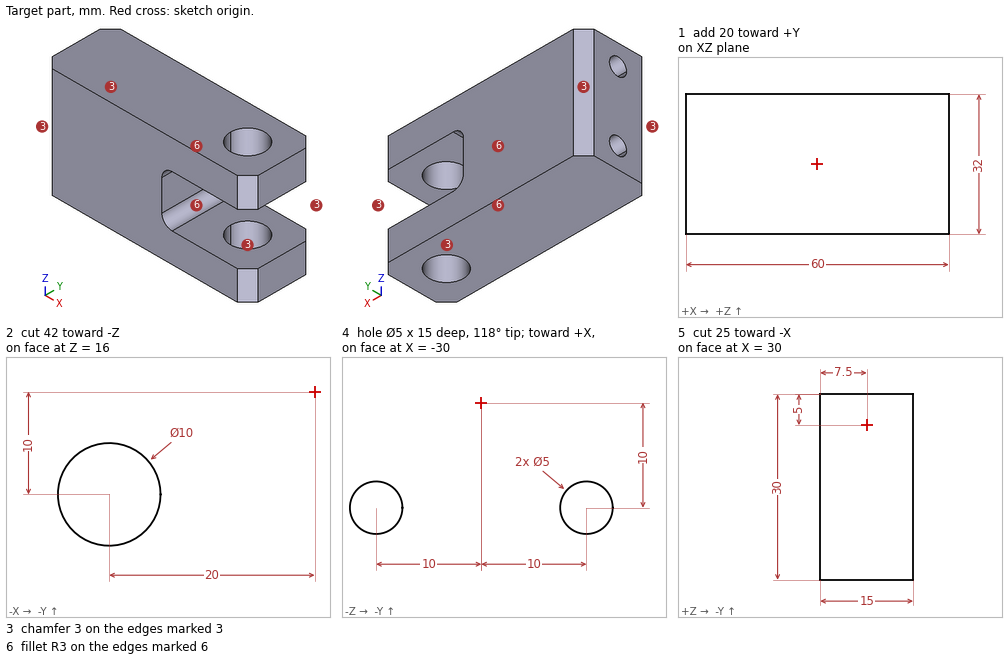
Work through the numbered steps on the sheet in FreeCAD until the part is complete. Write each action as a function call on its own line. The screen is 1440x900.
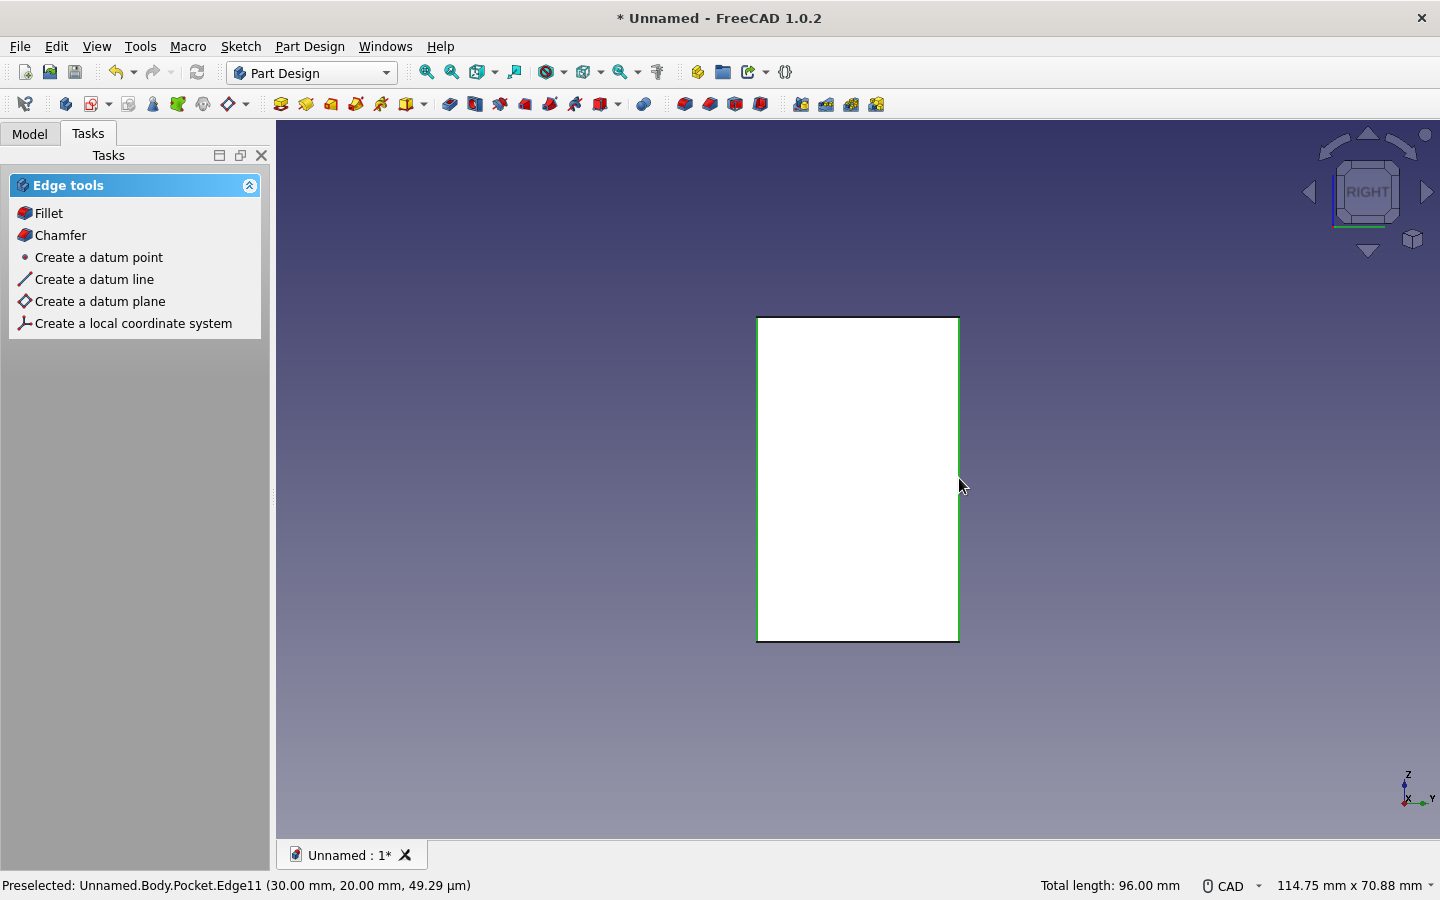
key(5)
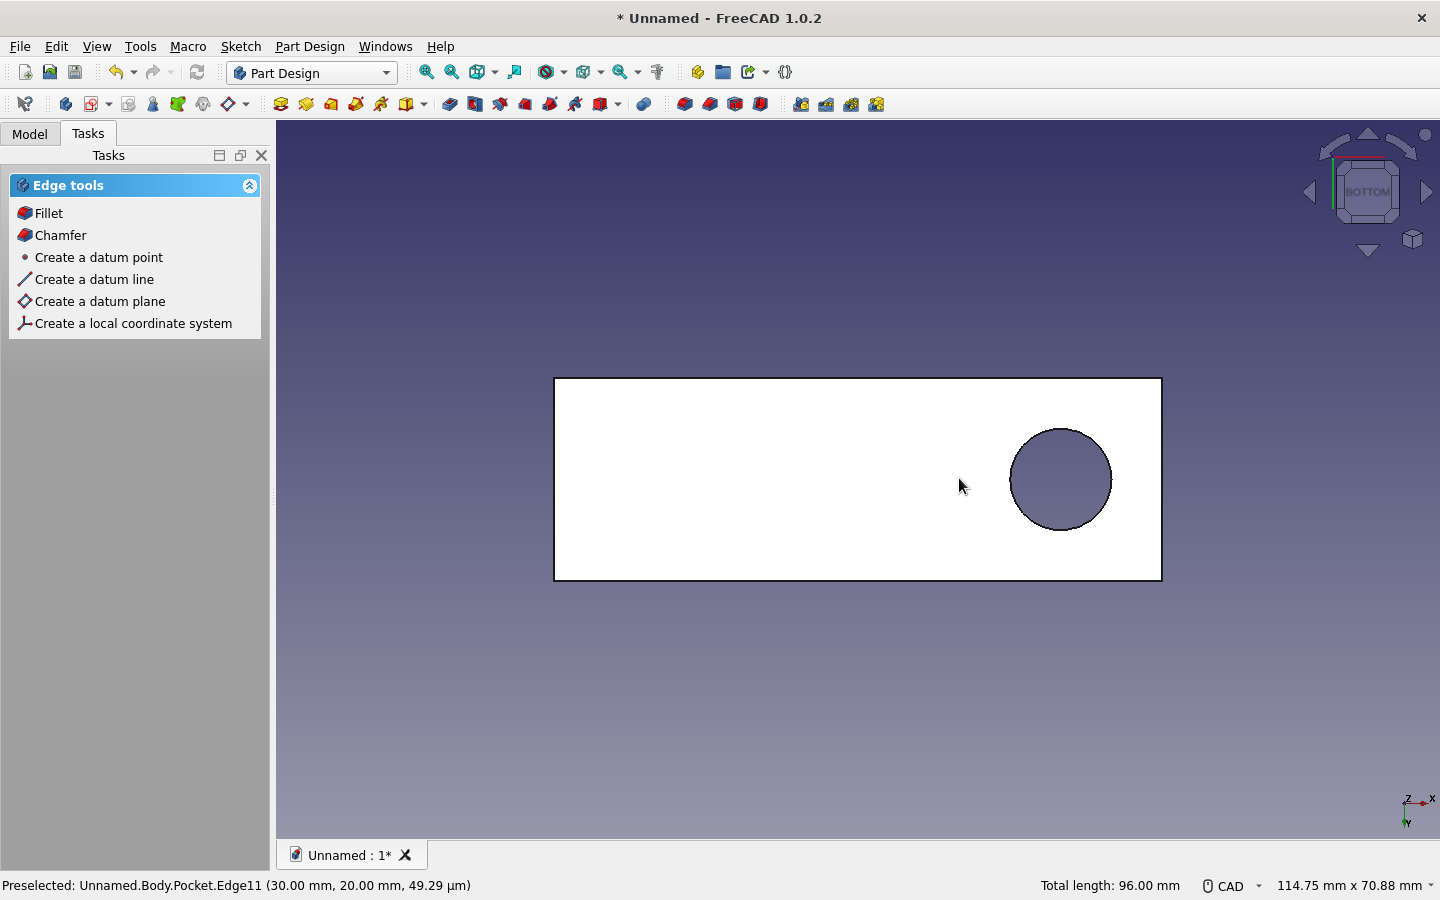
key(4)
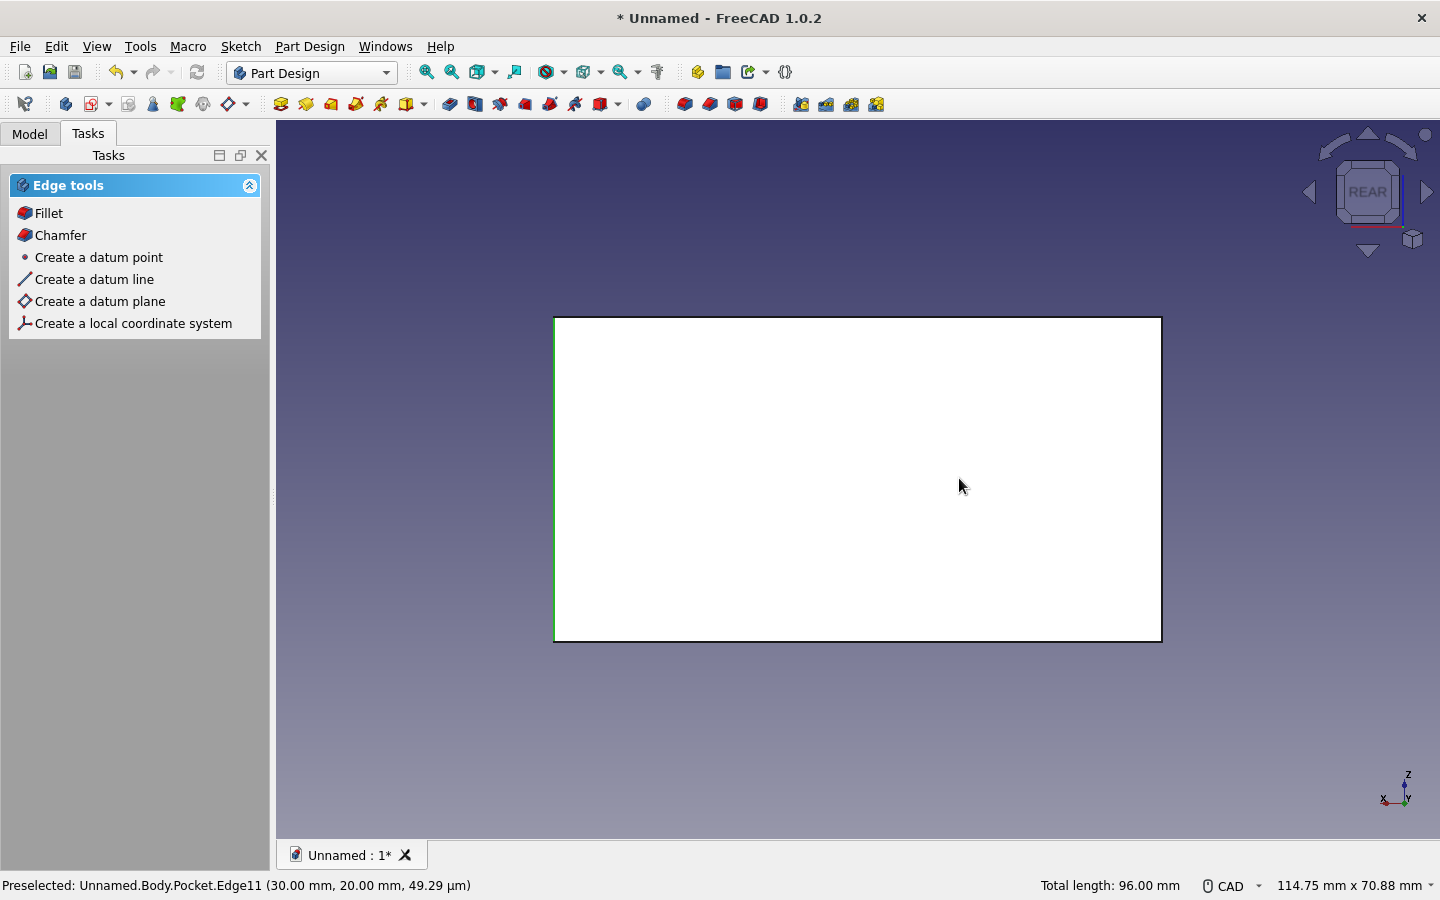
click(1162, 478, ctrl)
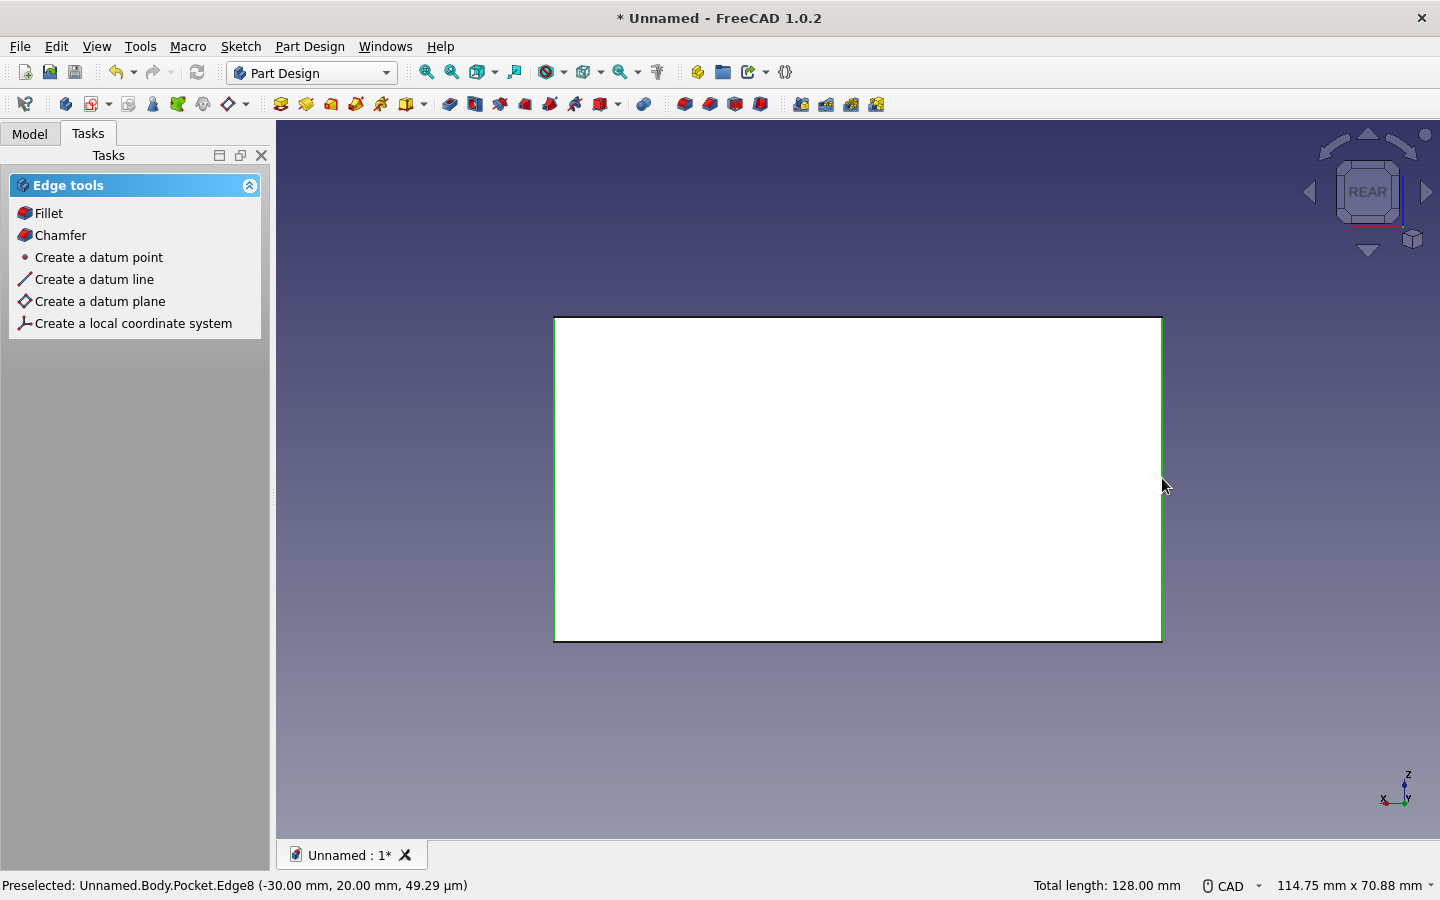
click(710, 104)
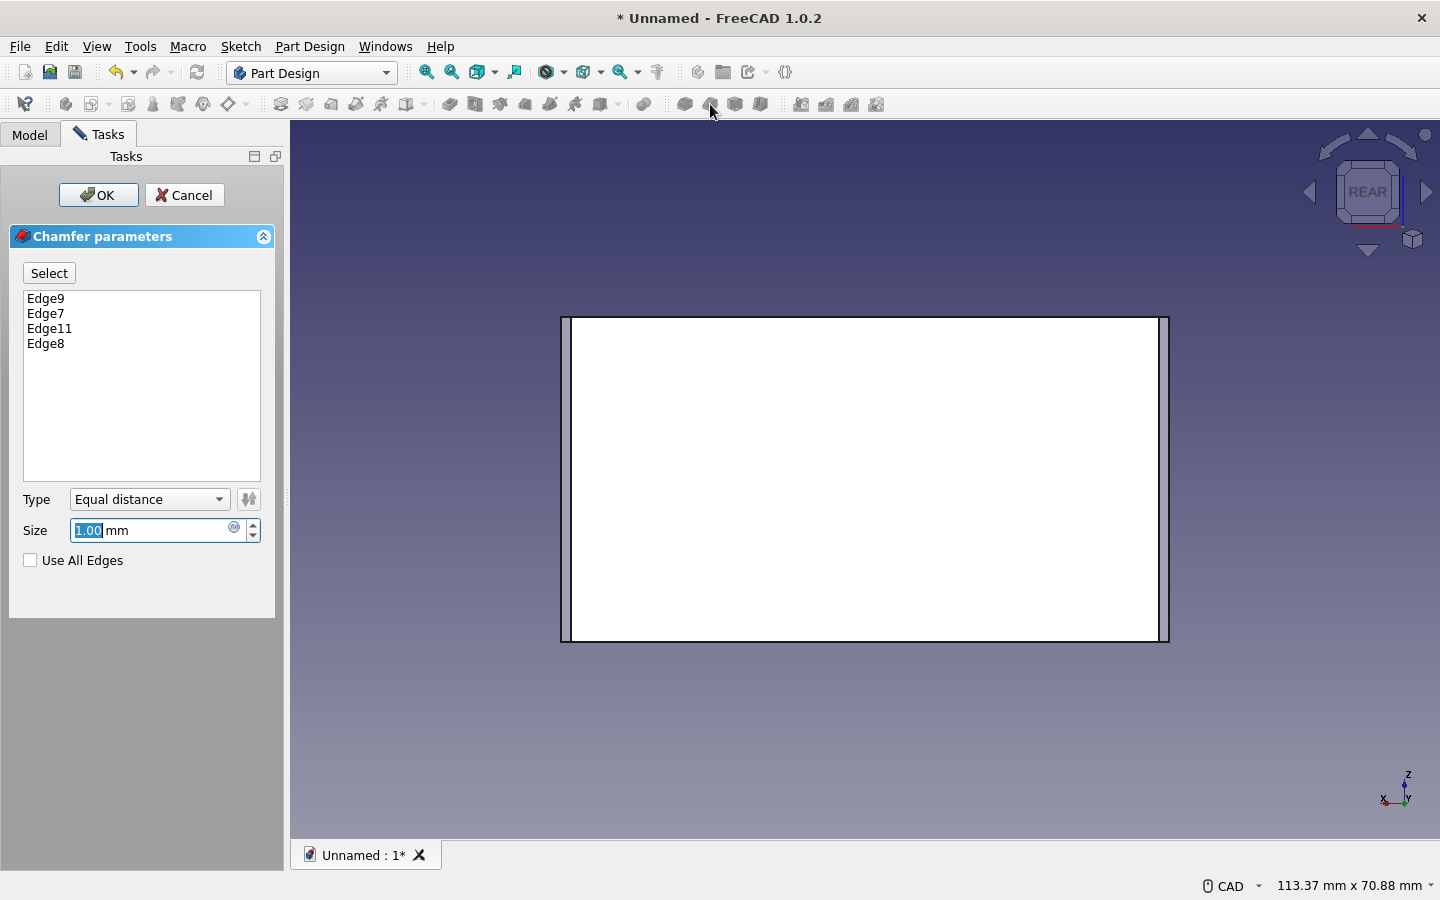
text(3)
key(Tab)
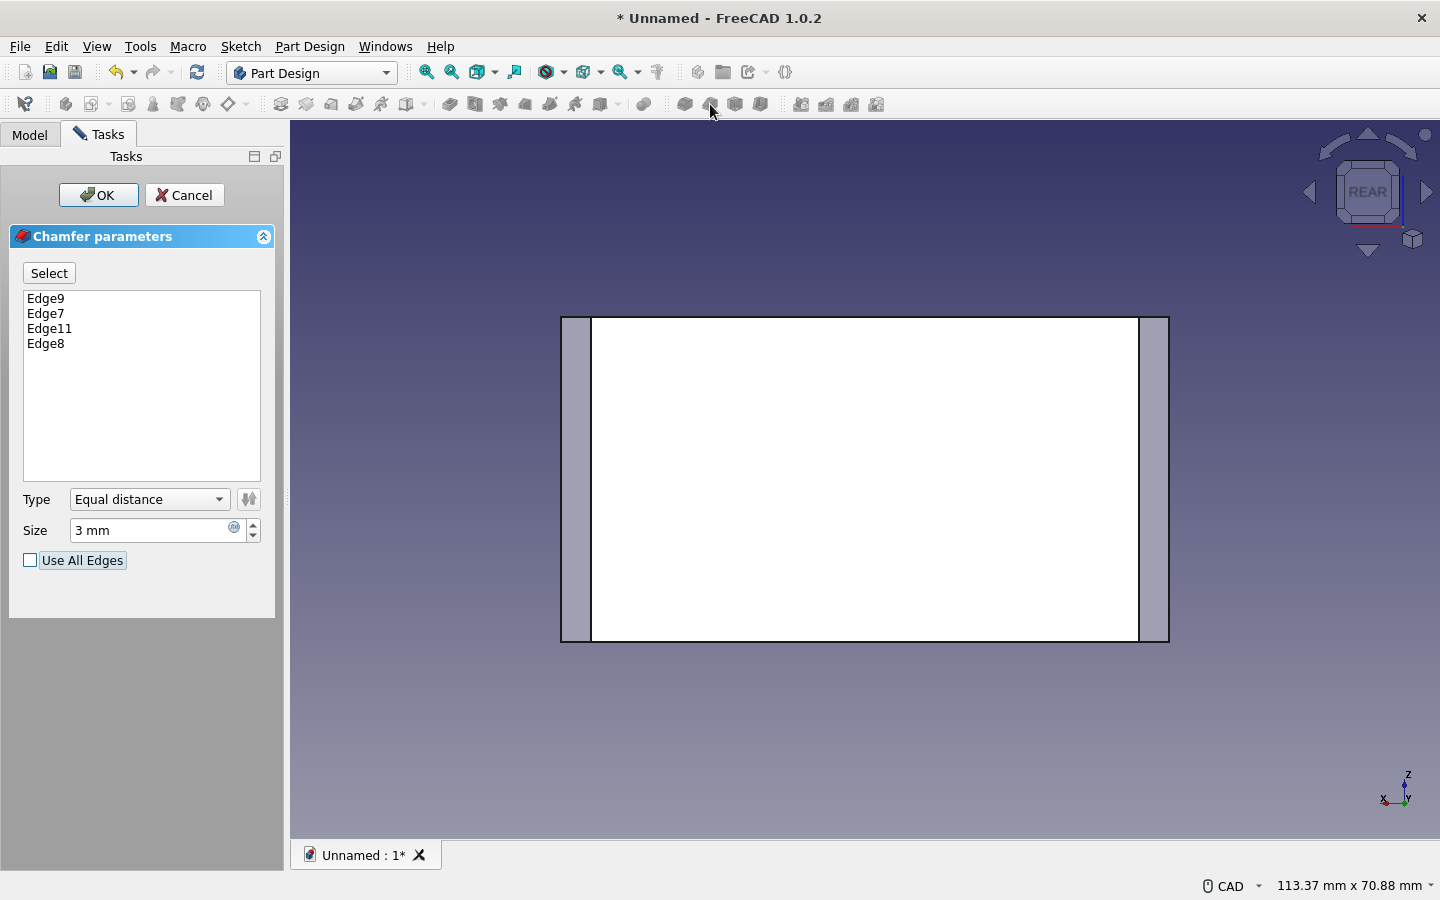
click(99, 195)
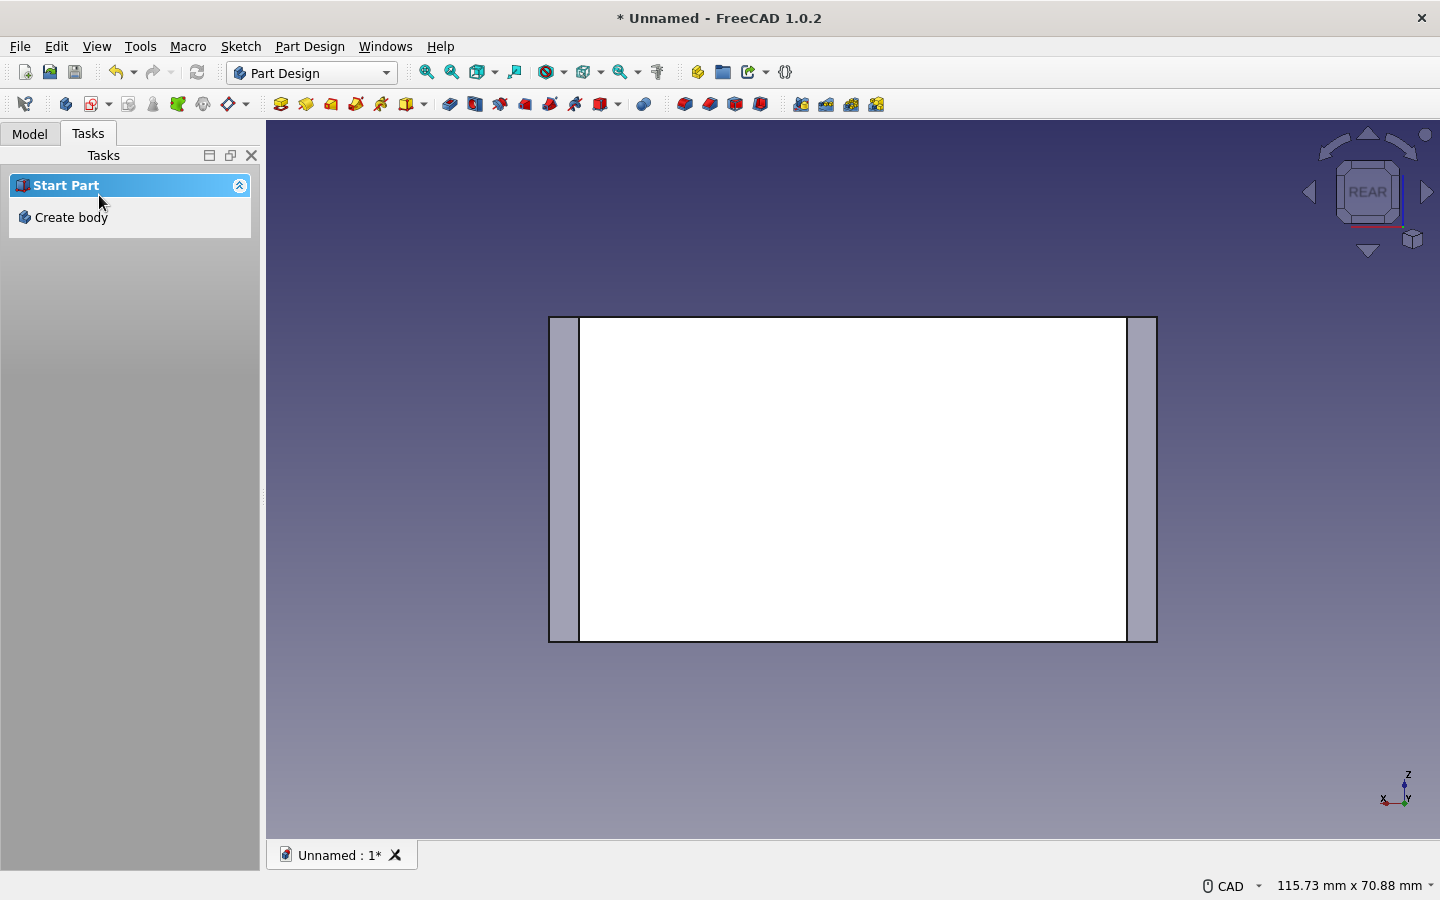
key(6)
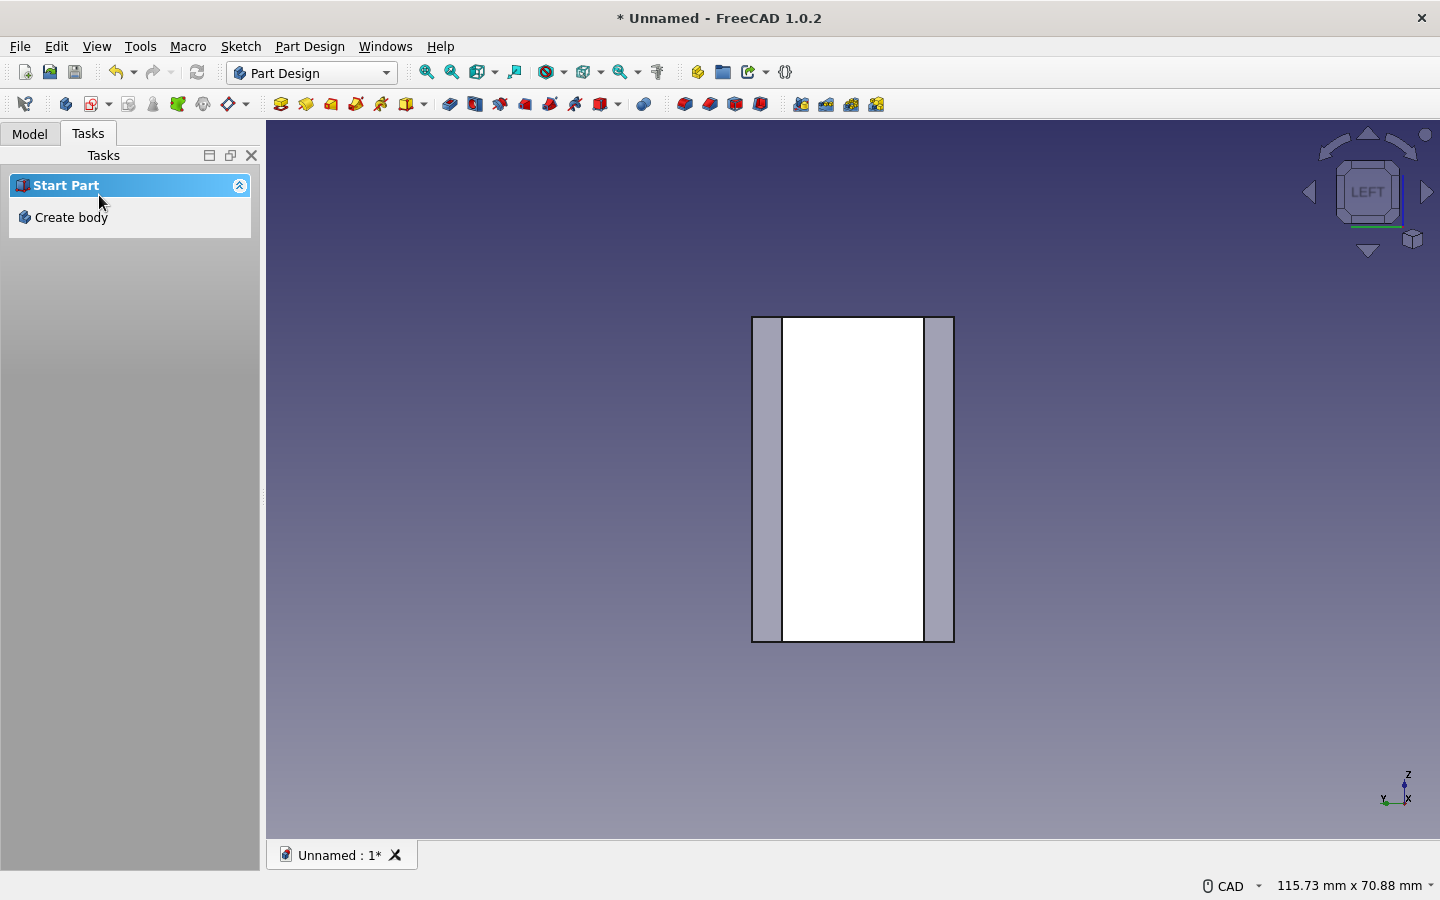
click(853, 432)